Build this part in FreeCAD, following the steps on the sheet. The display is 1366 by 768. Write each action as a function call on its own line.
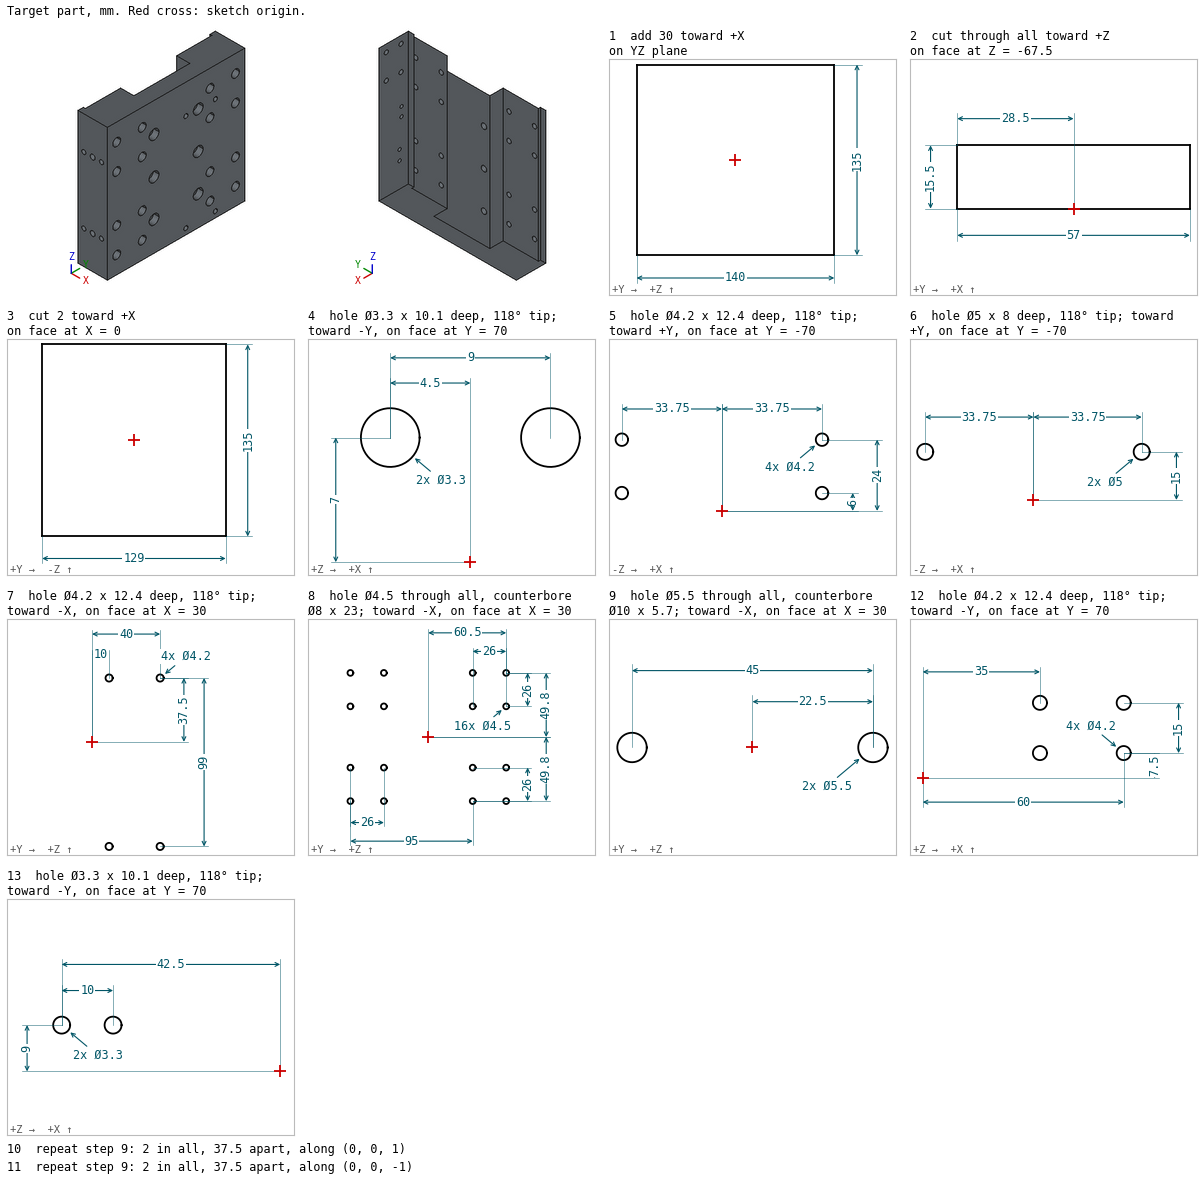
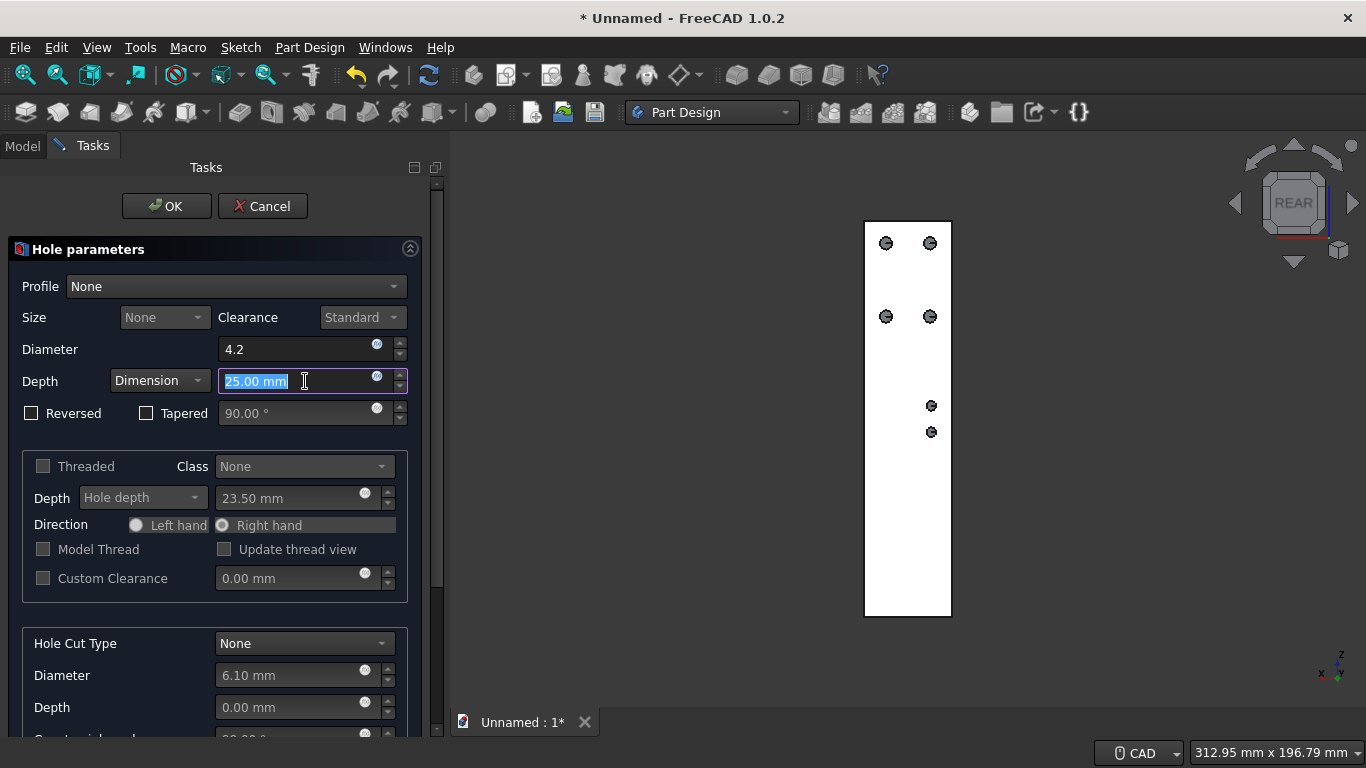
text(12.4)
key(Tab)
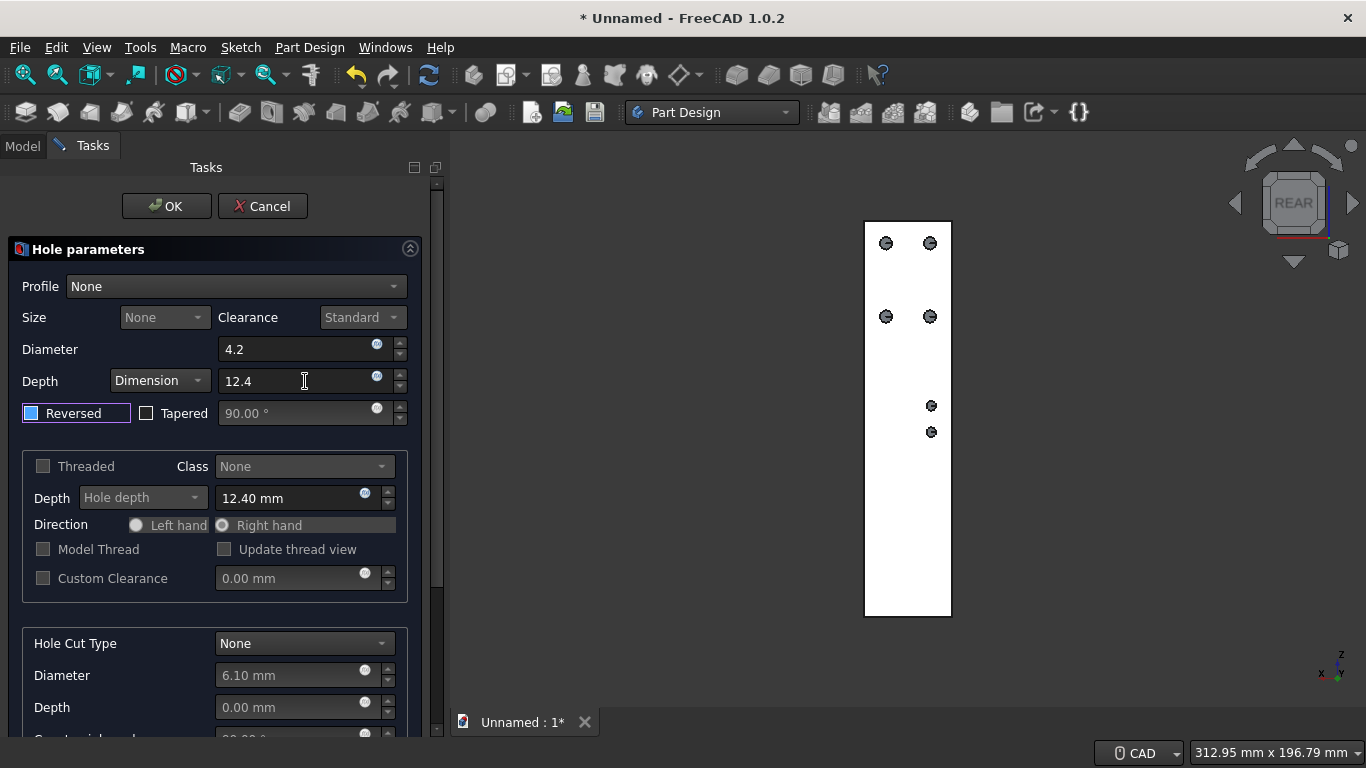
click(167, 206)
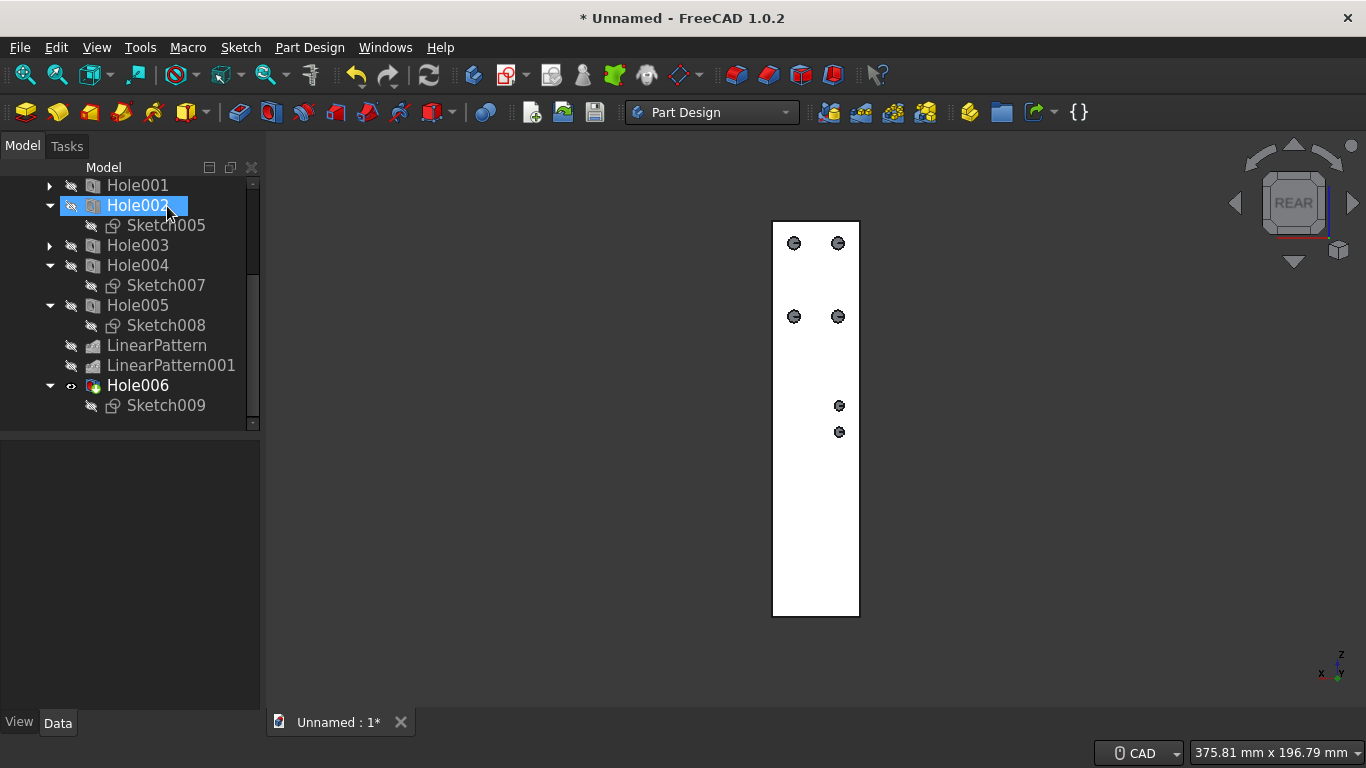
click(816, 531)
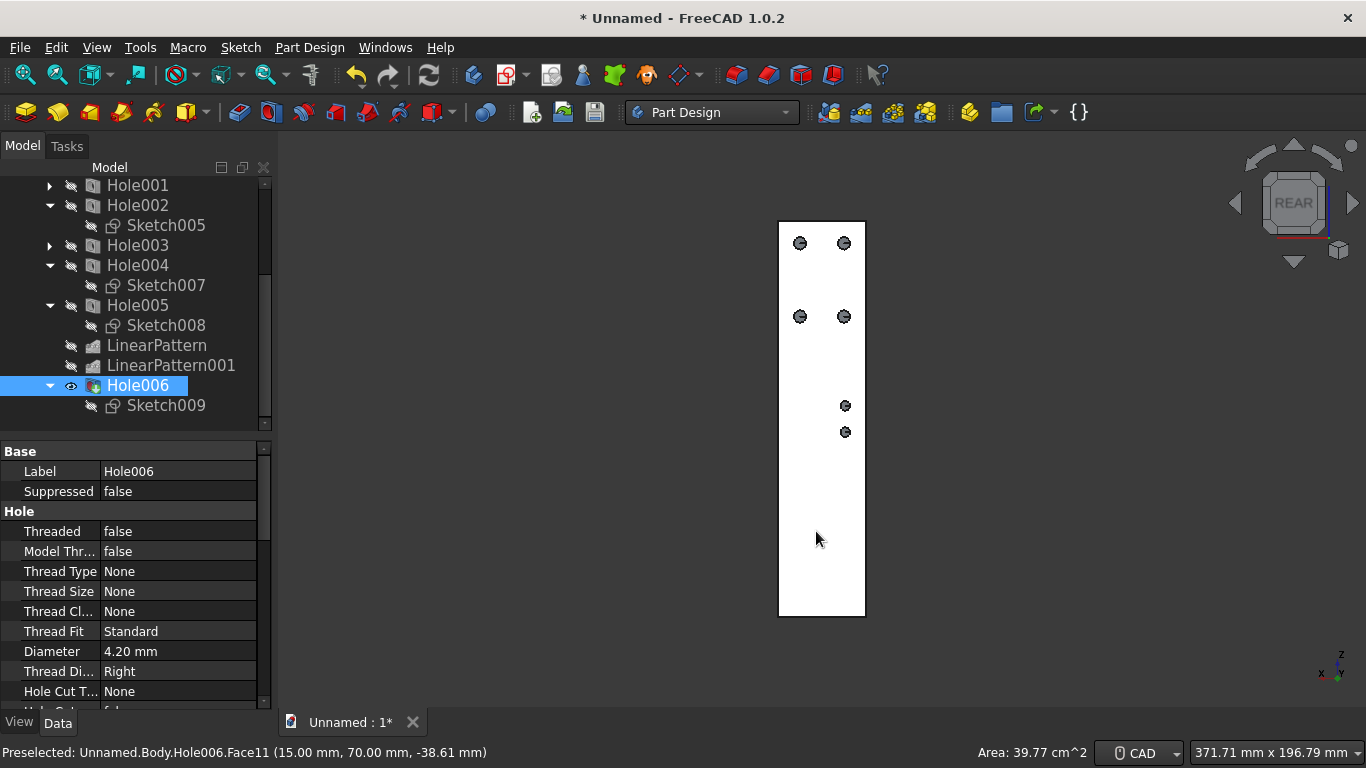
click(506, 76)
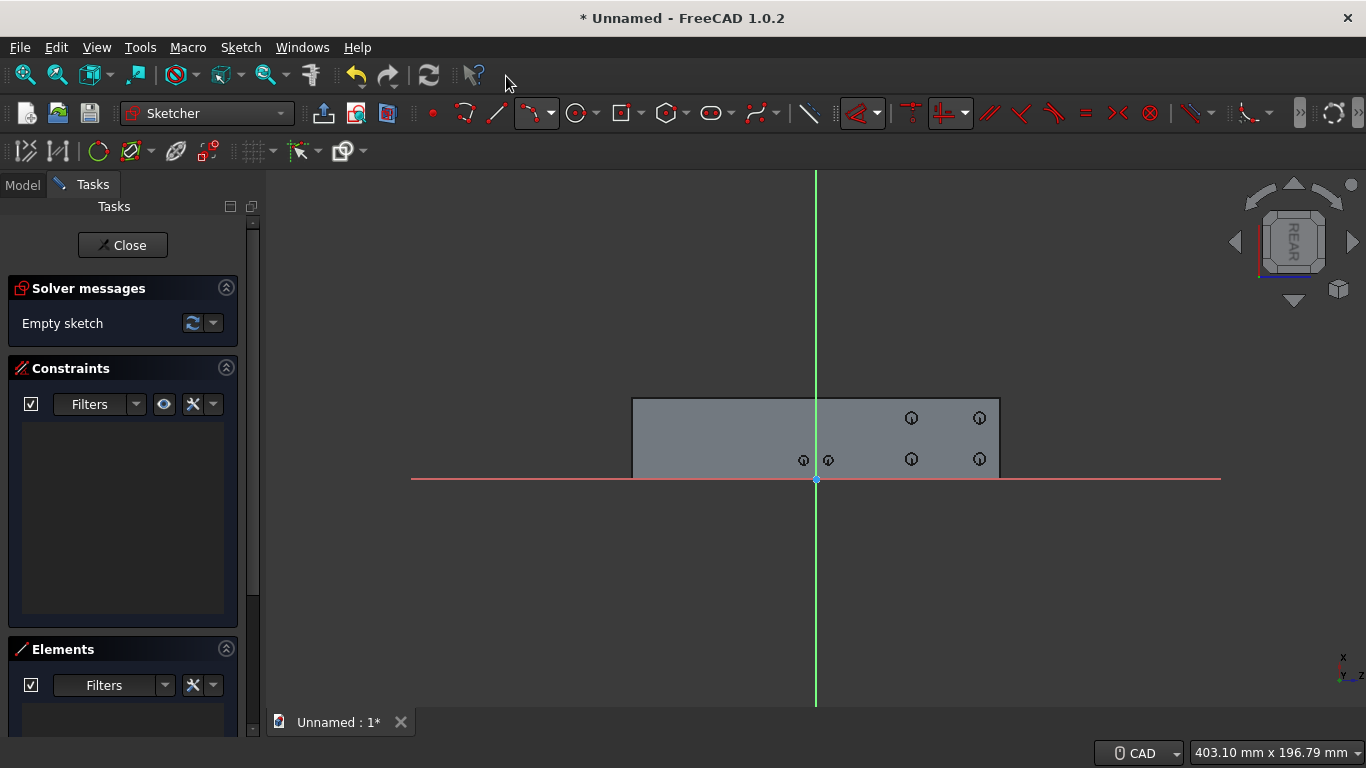
scroll(711, 456, up, 14)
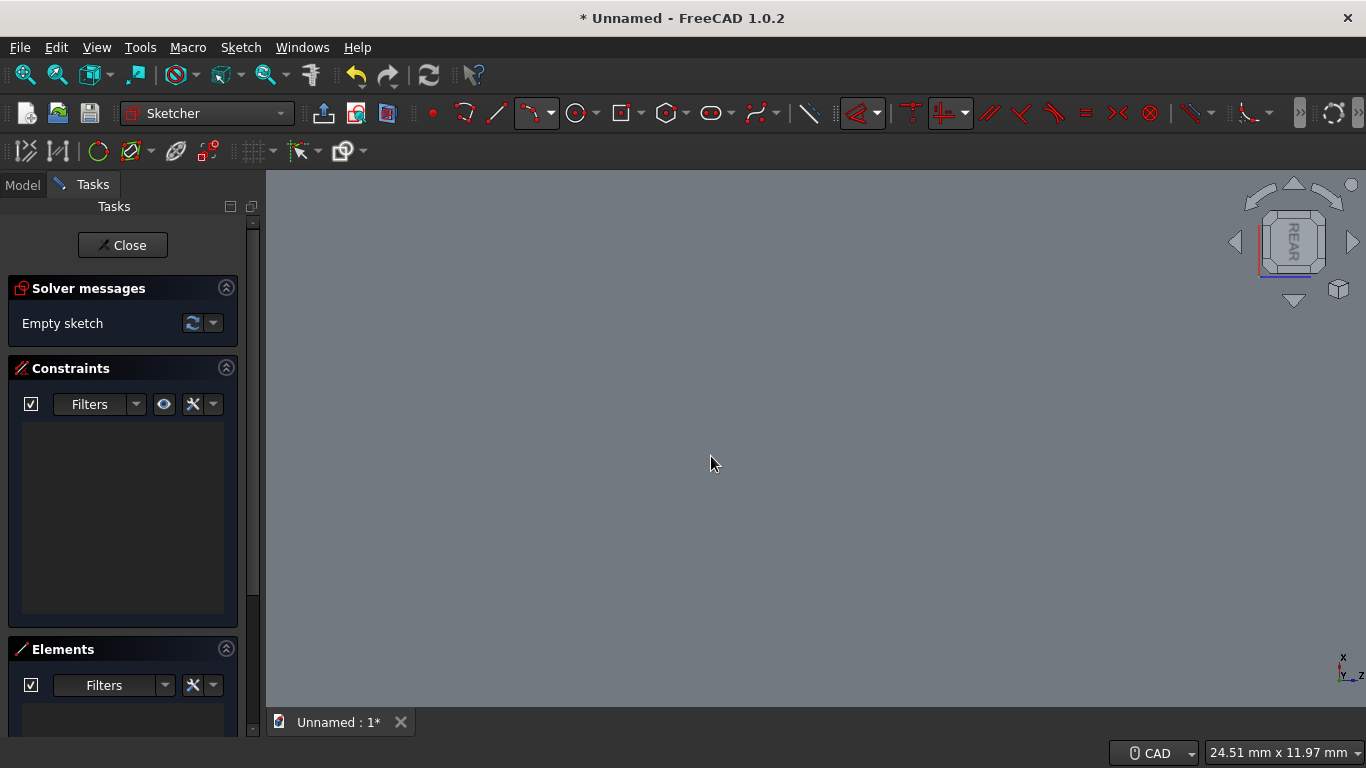
click(576, 114)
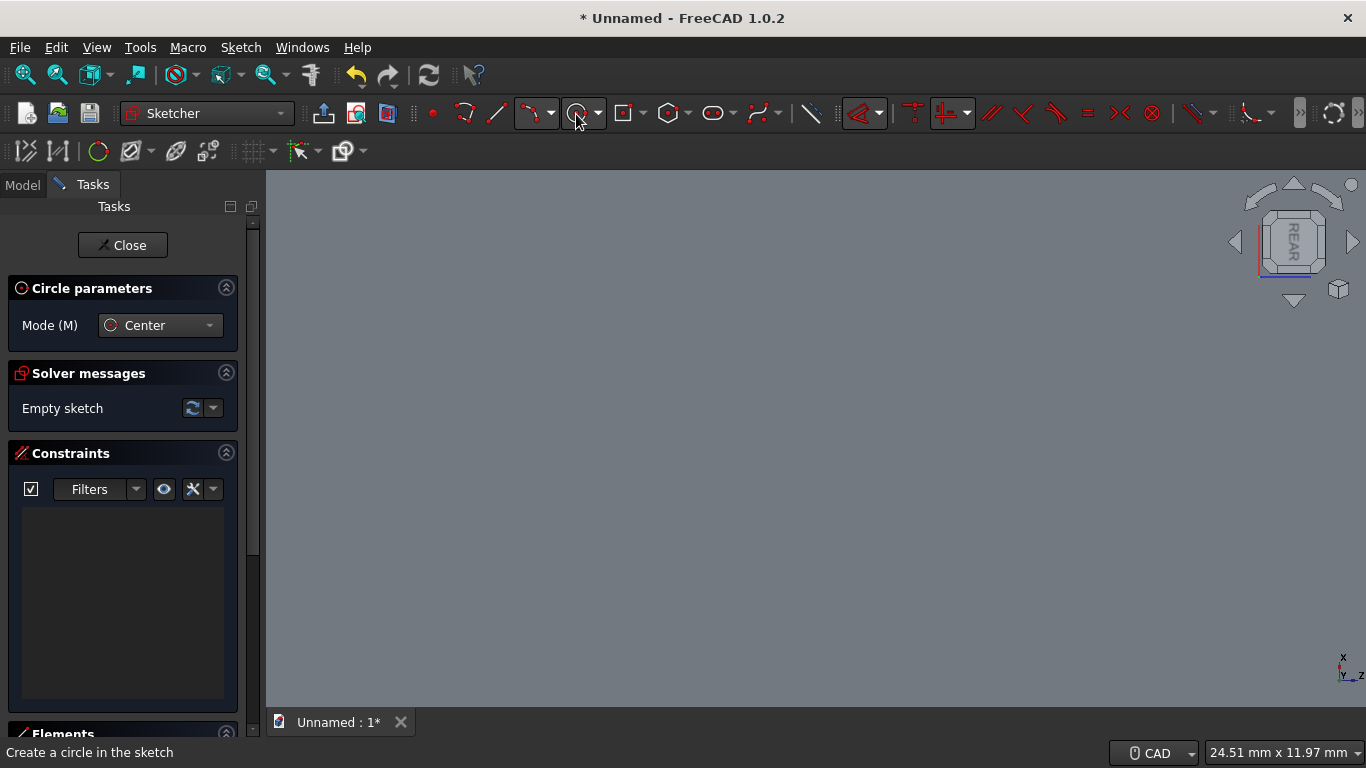
click(524, 429)
click(577, 377)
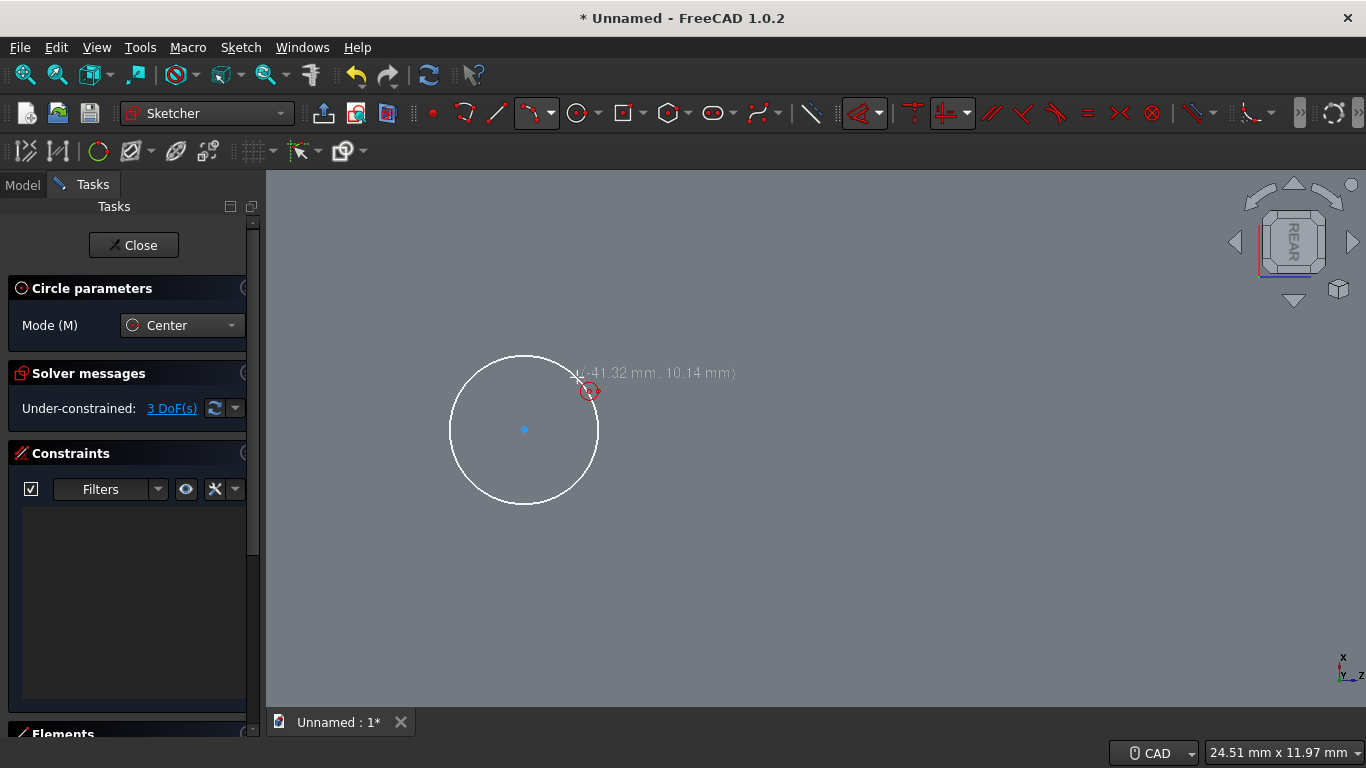
click(973, 429)
click(1025, 377)
key(Escape)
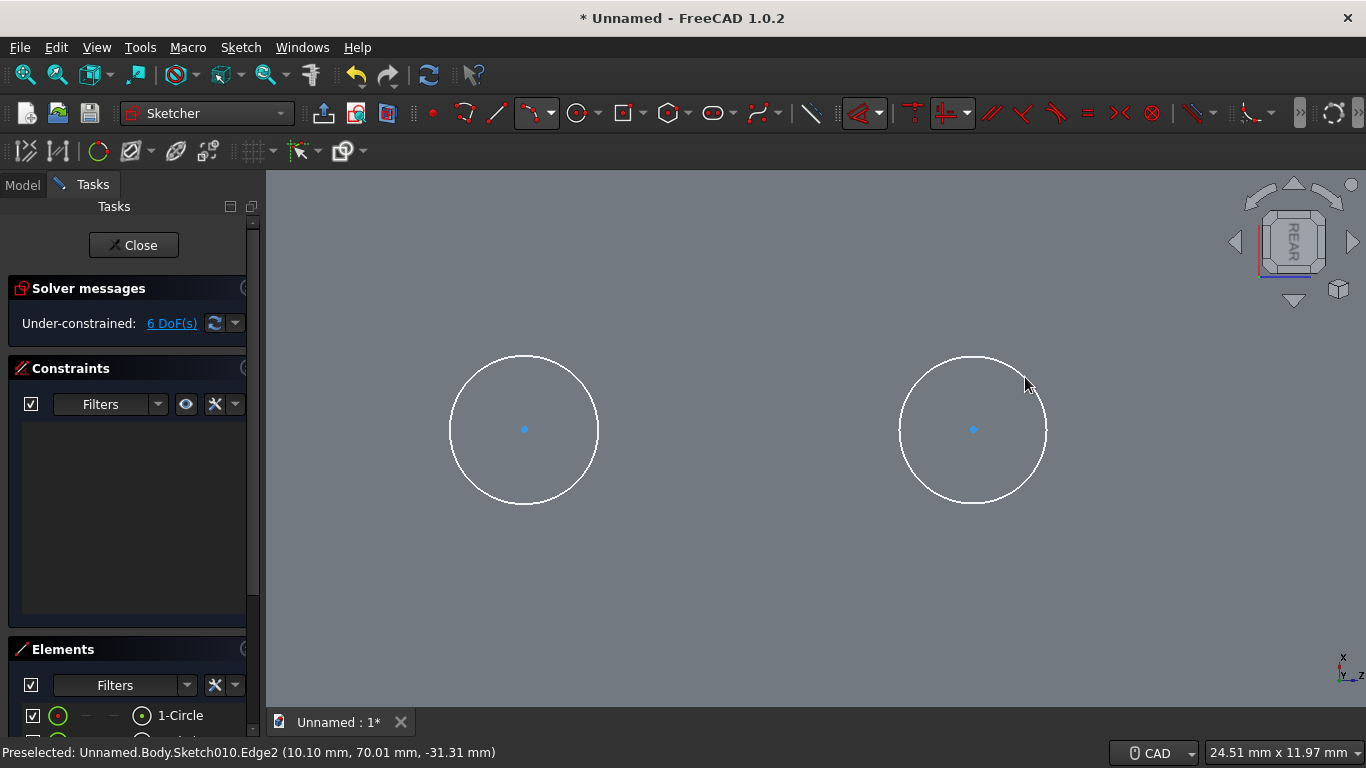
click(576, 377)